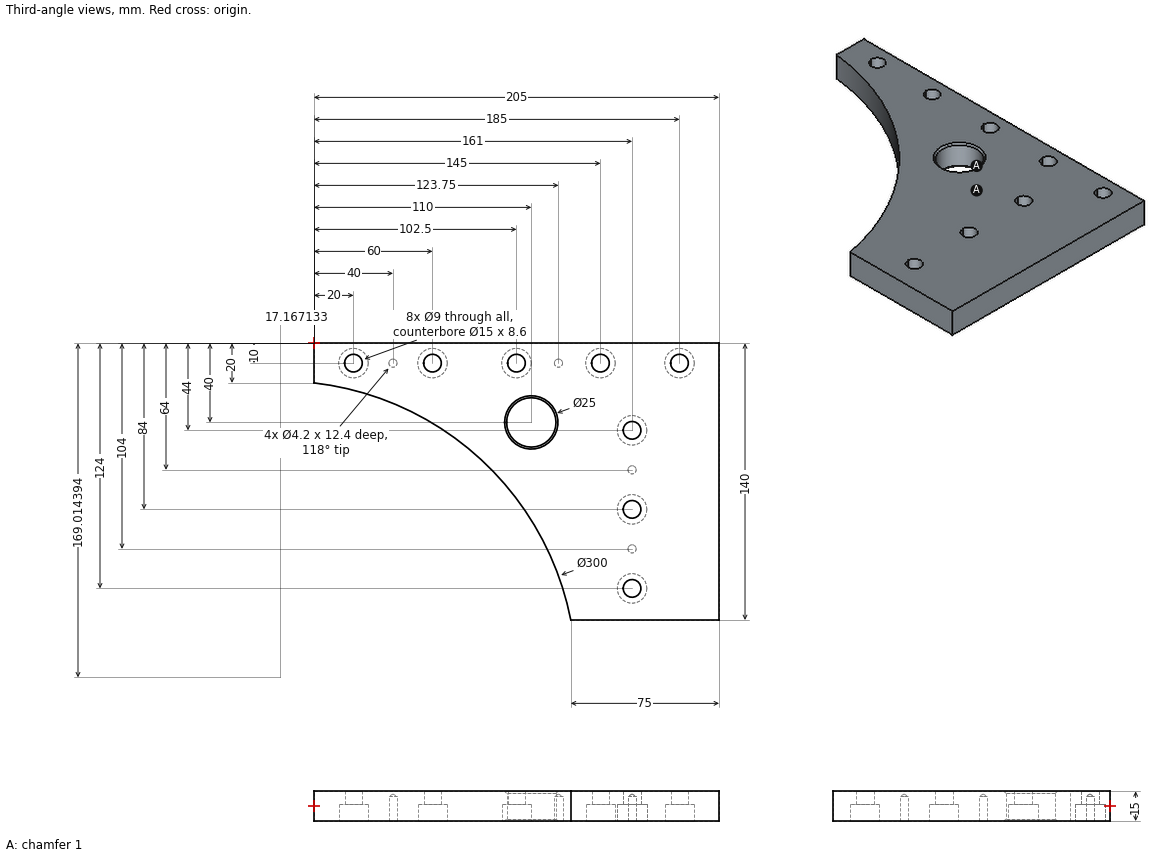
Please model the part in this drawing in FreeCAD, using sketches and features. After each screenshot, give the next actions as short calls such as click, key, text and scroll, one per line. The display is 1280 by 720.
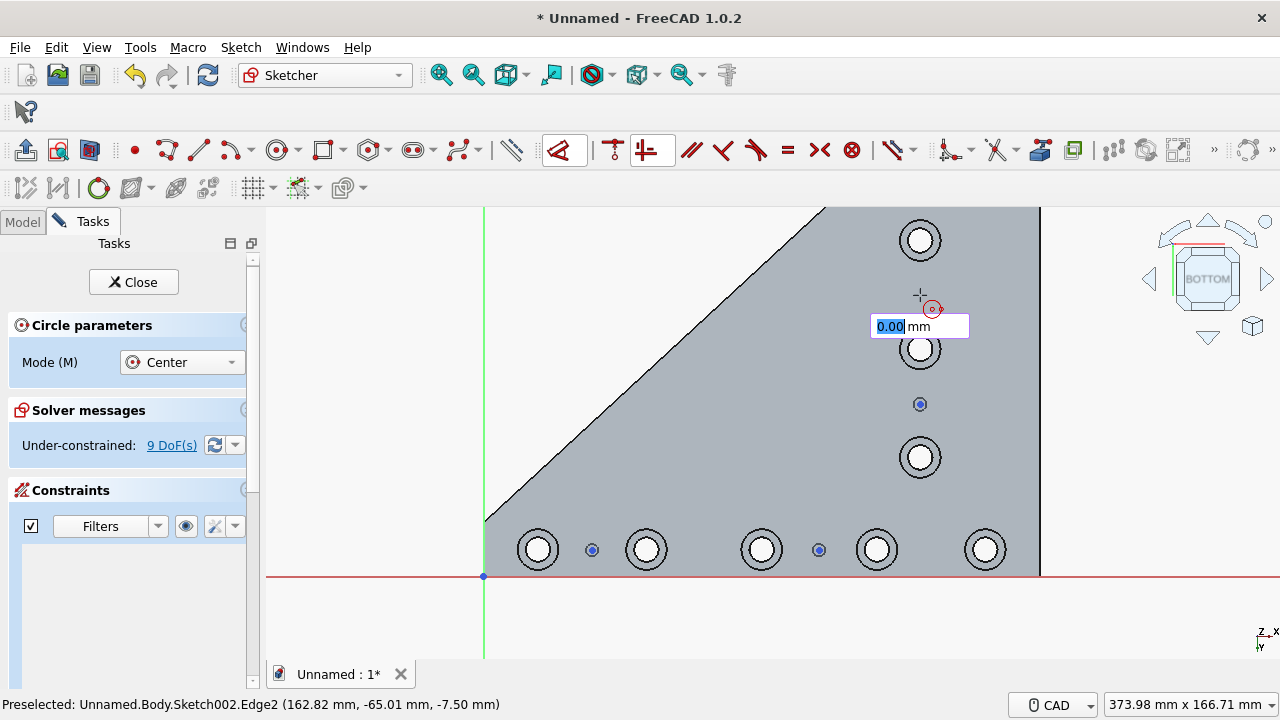
scroll(924, 291, up, 6)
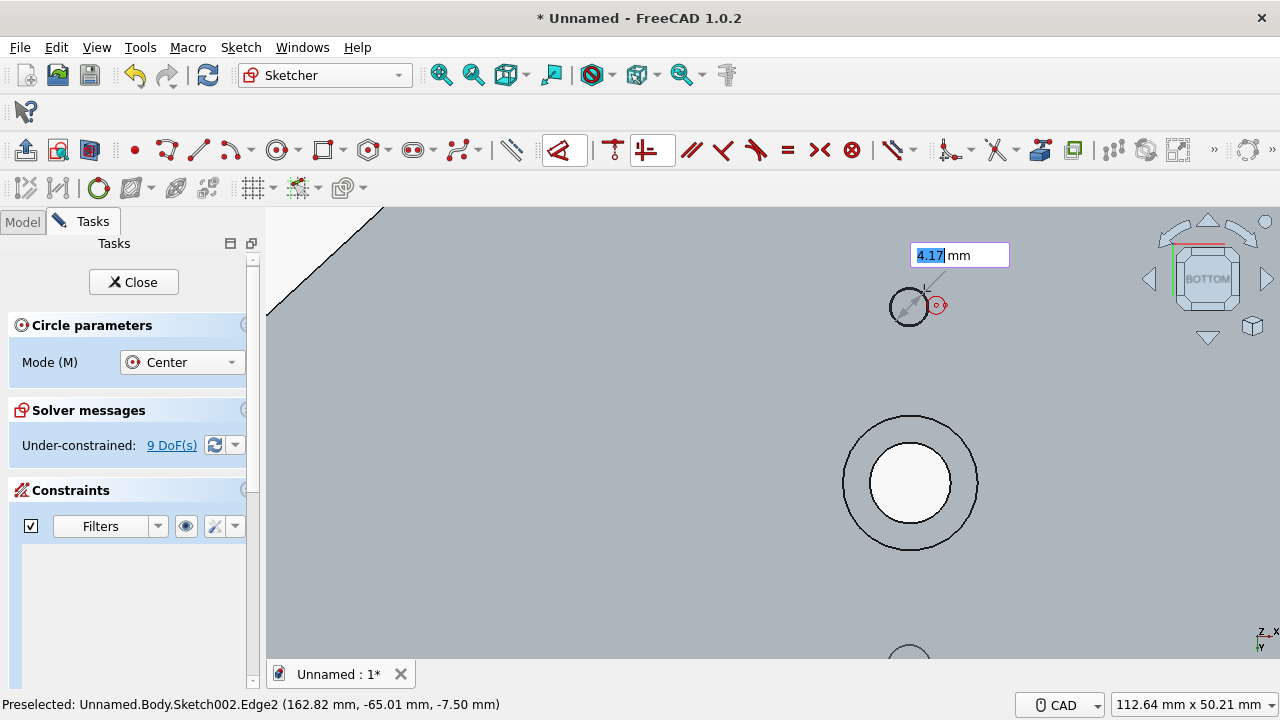
click(924, 290)
key(Escape)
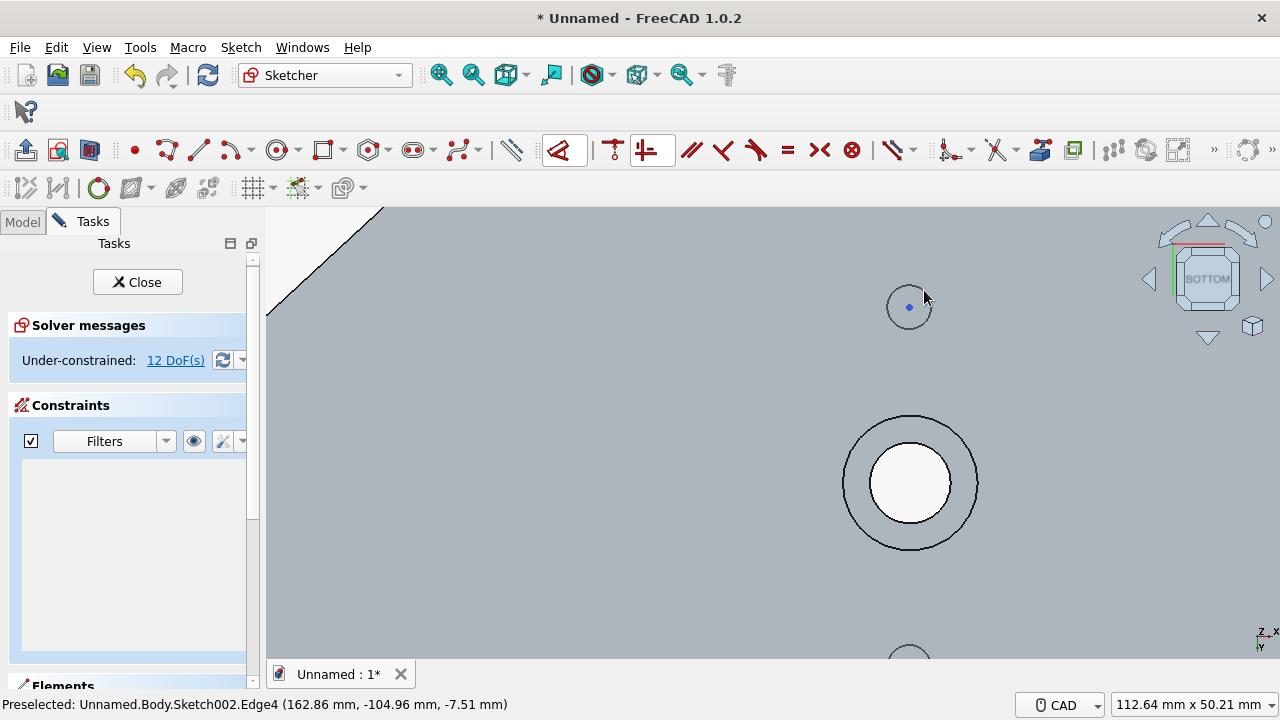
scroll(924, 291, down, 6)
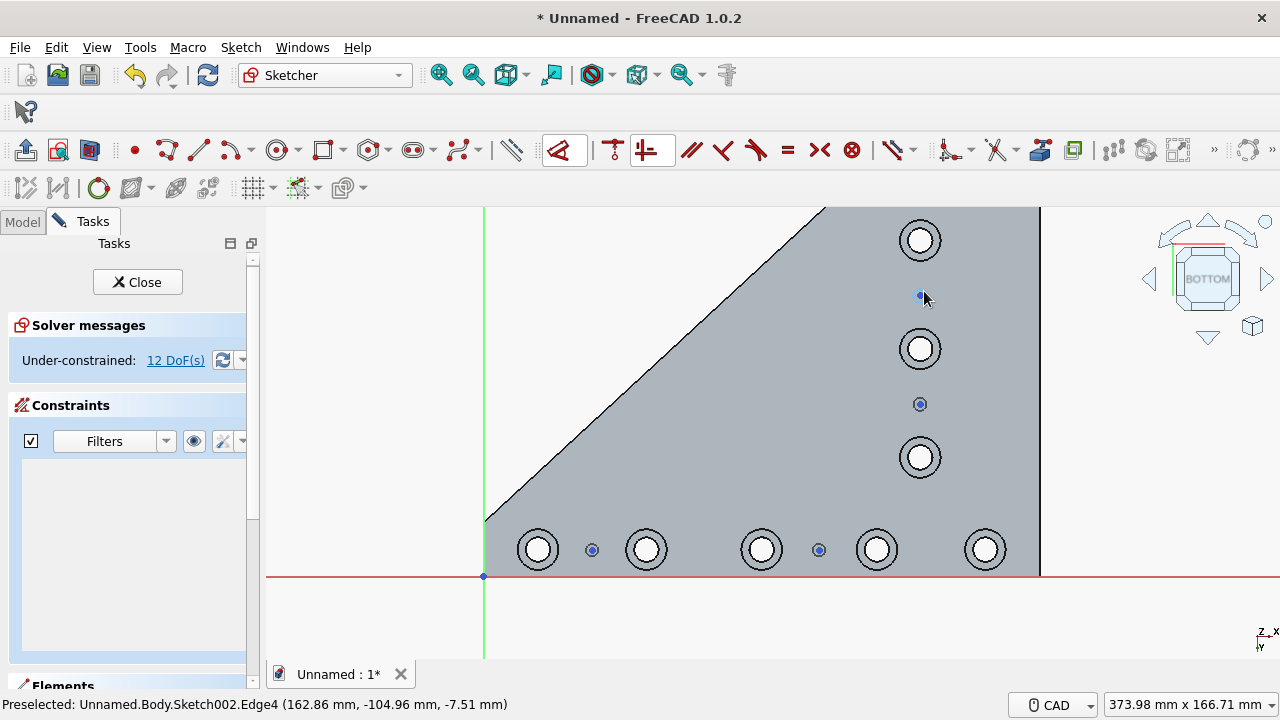
scroll(596, 546, up, 5)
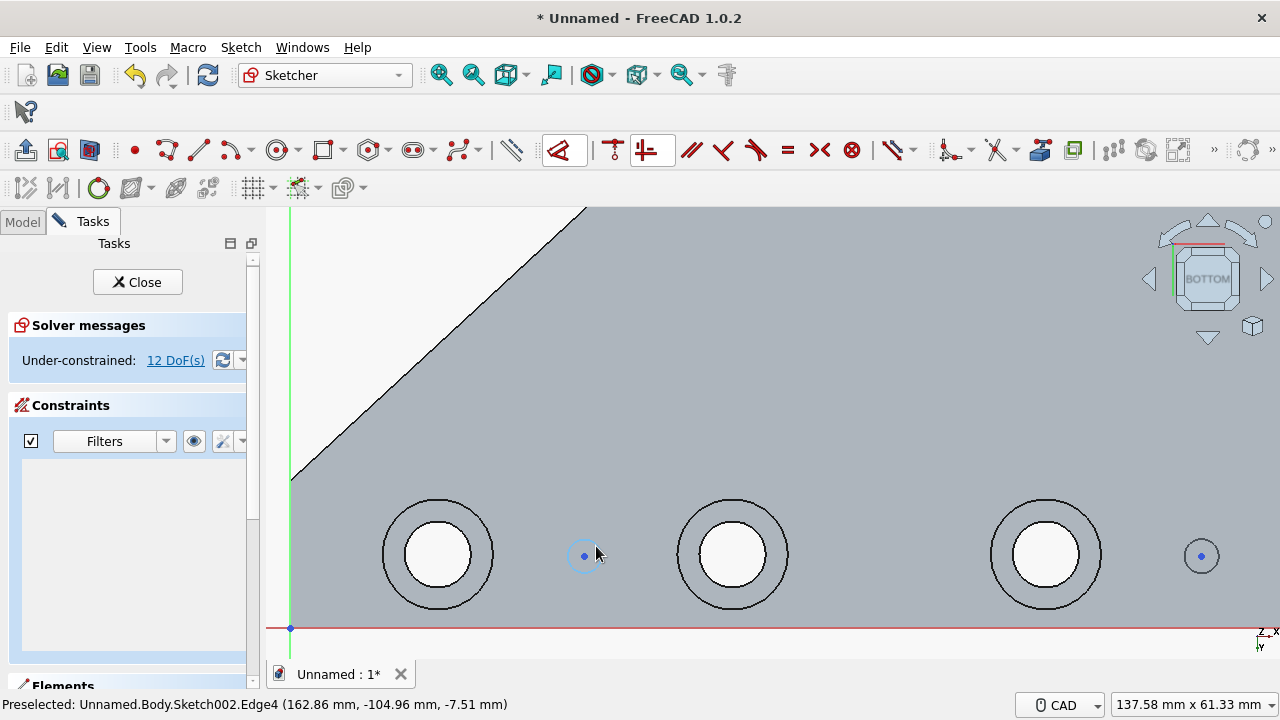
click(596, 544)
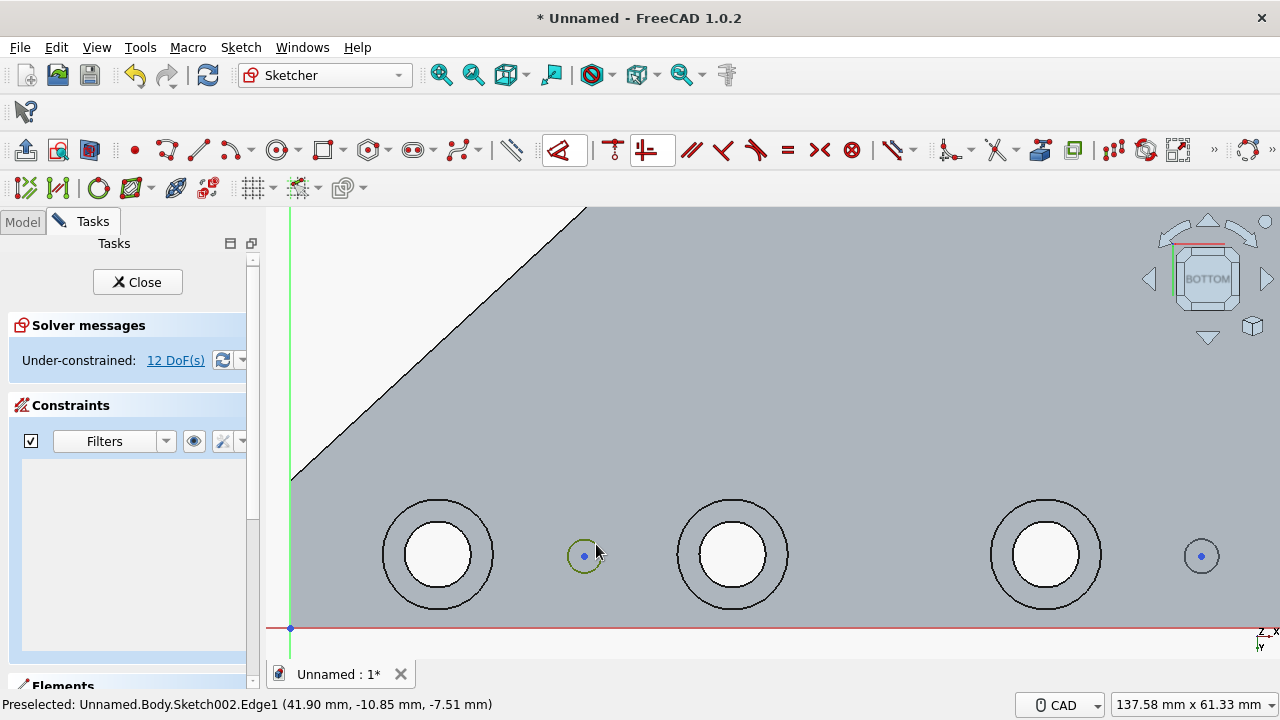
scroll(596, 547, down, 5)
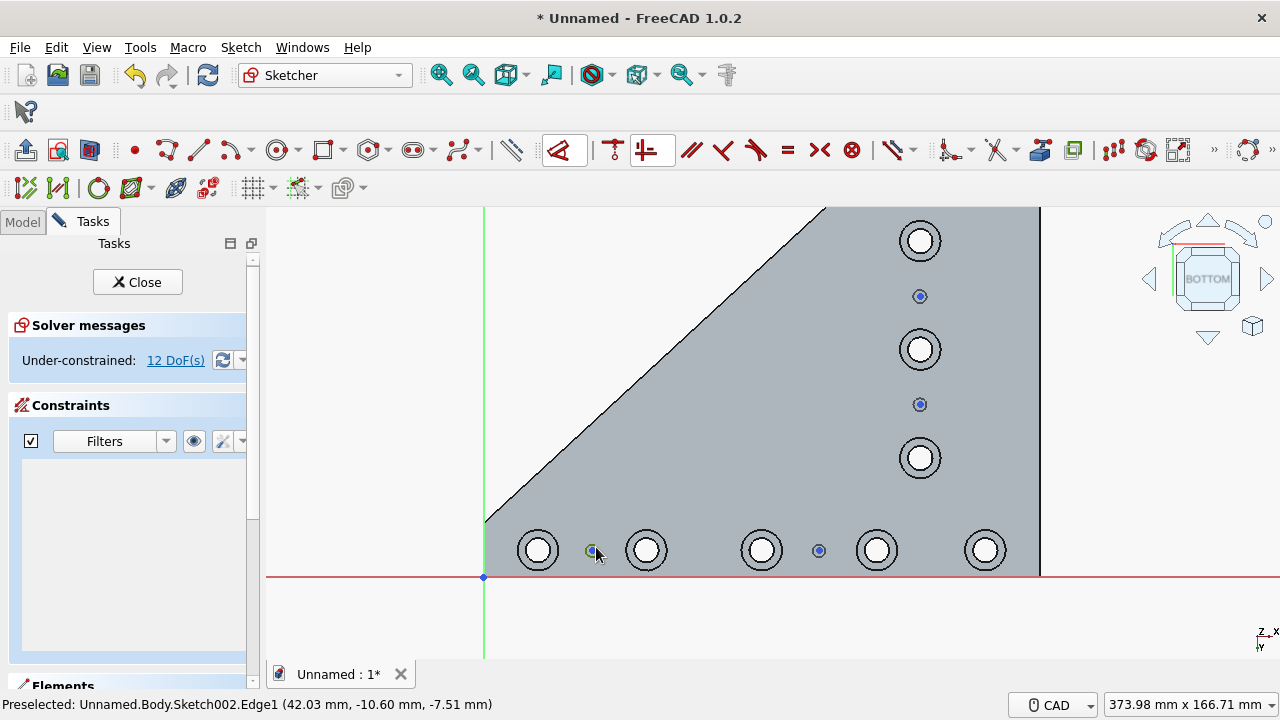
scroll(823, 546, up, 4)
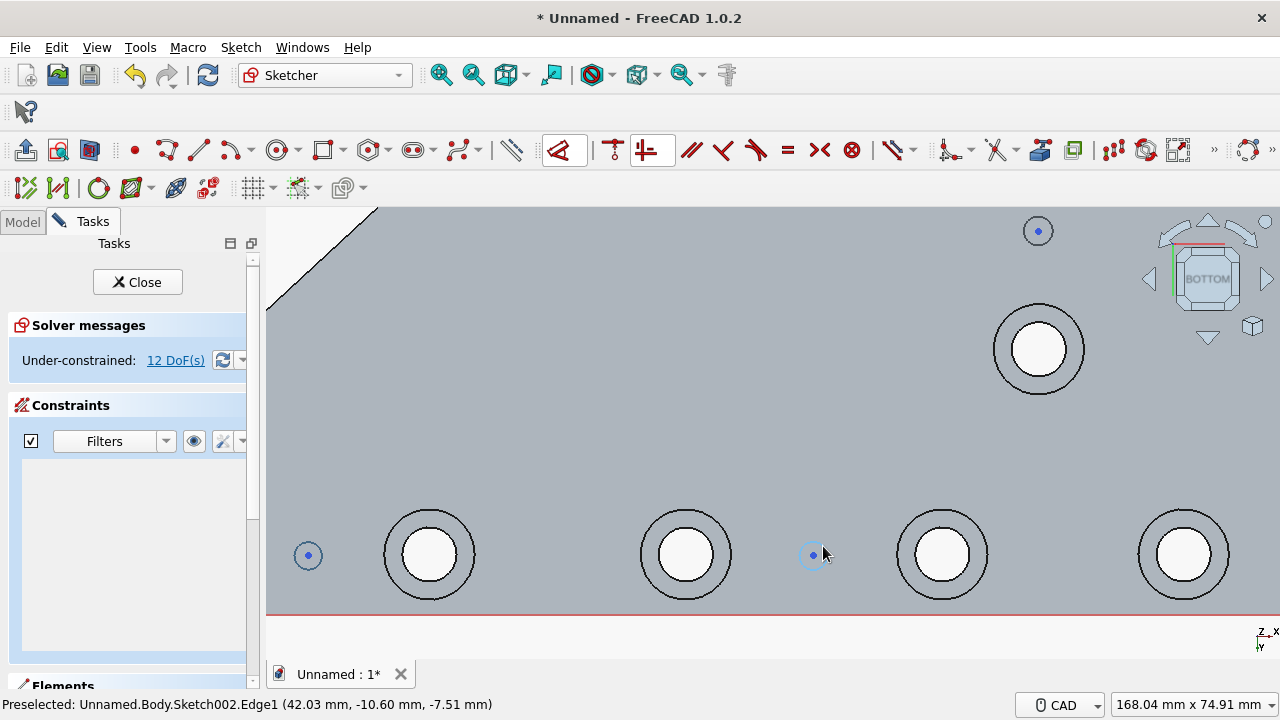
click(823, 546)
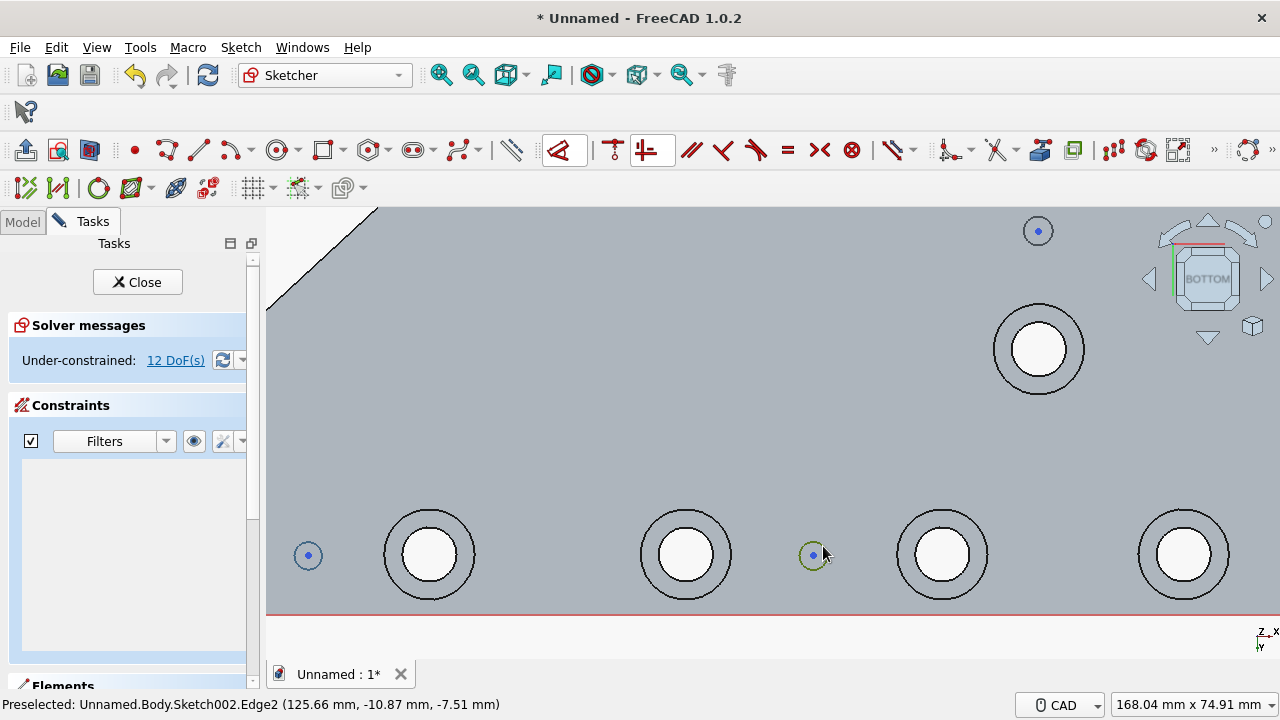
click(1028, 241)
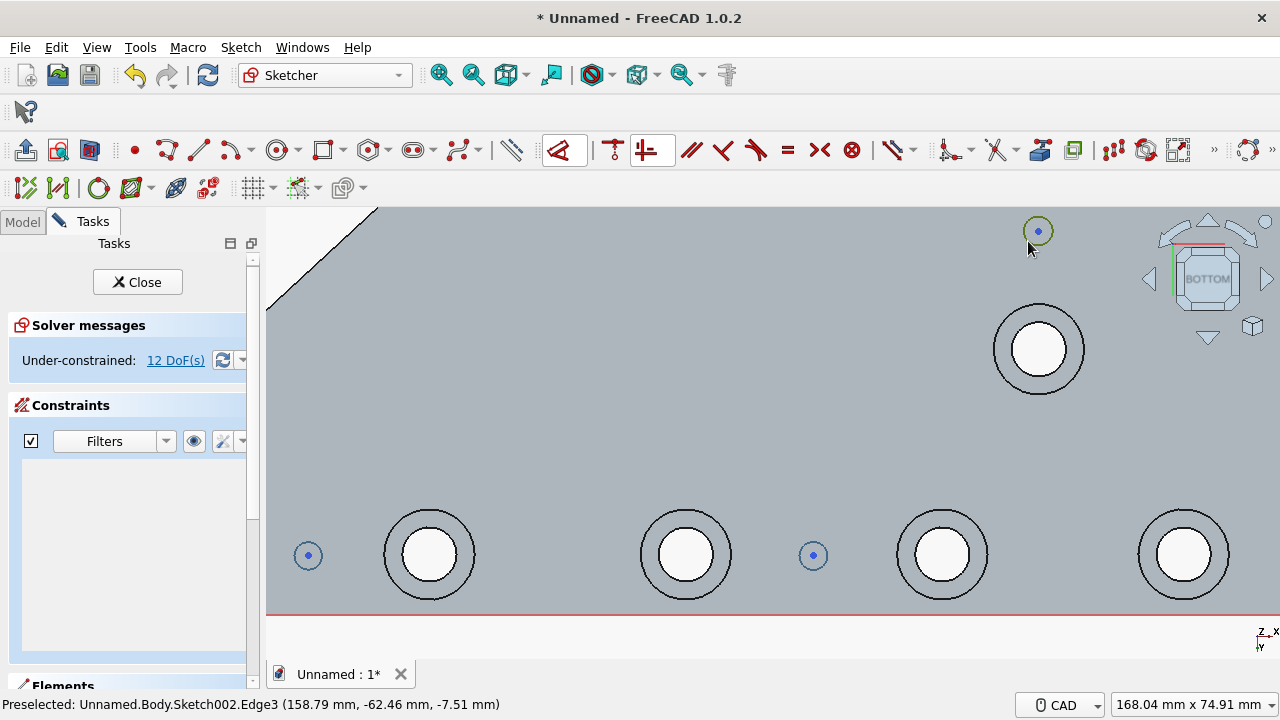
scroll(823, 546, down, 4)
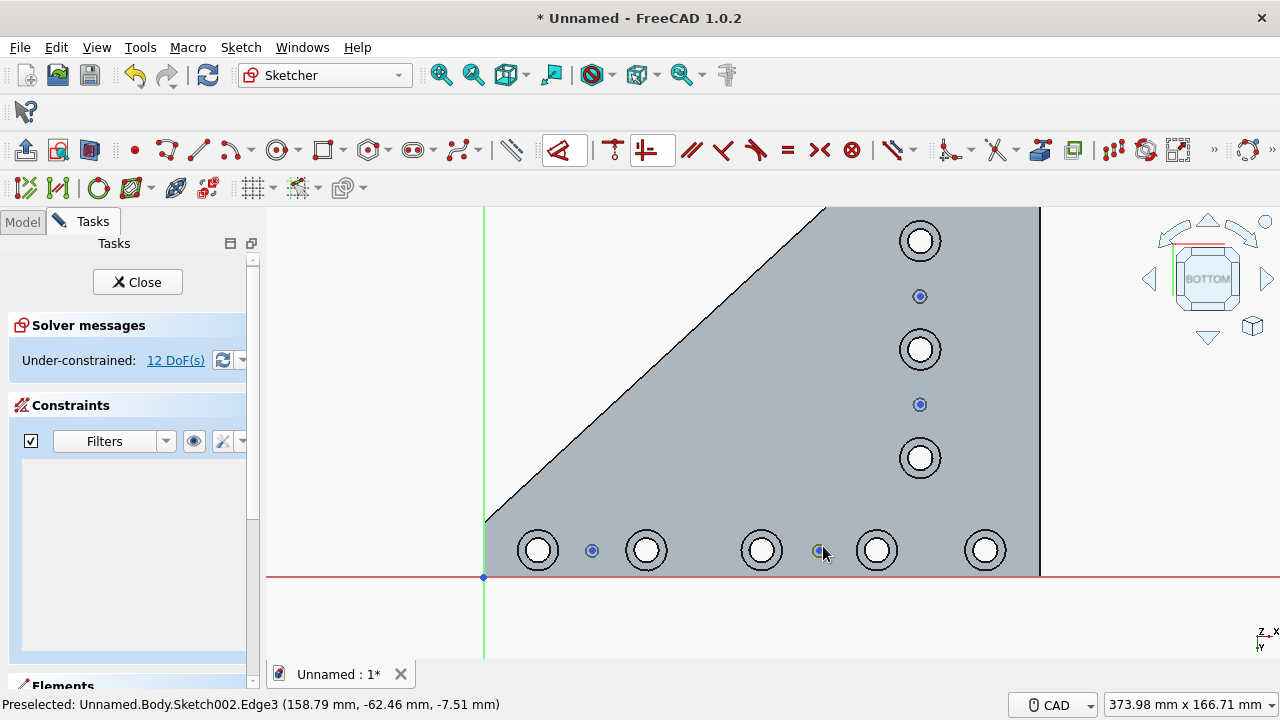
scroll(925, 292, up, 4)